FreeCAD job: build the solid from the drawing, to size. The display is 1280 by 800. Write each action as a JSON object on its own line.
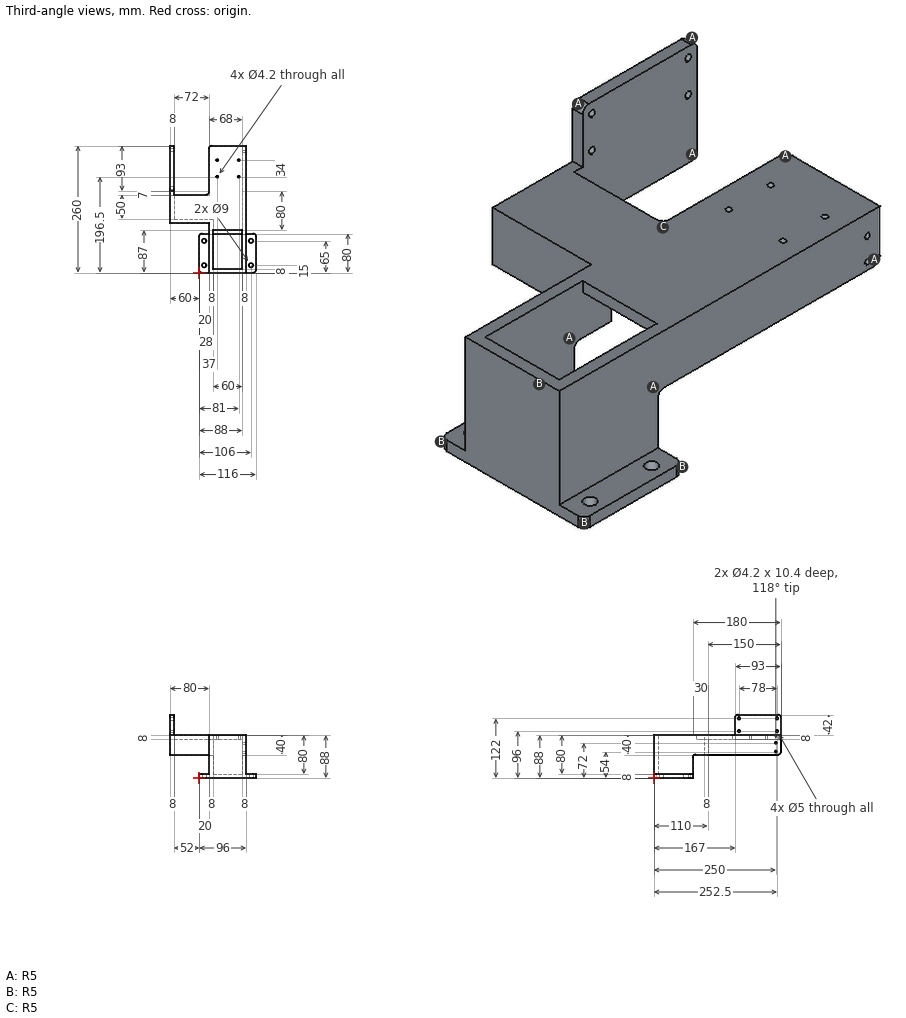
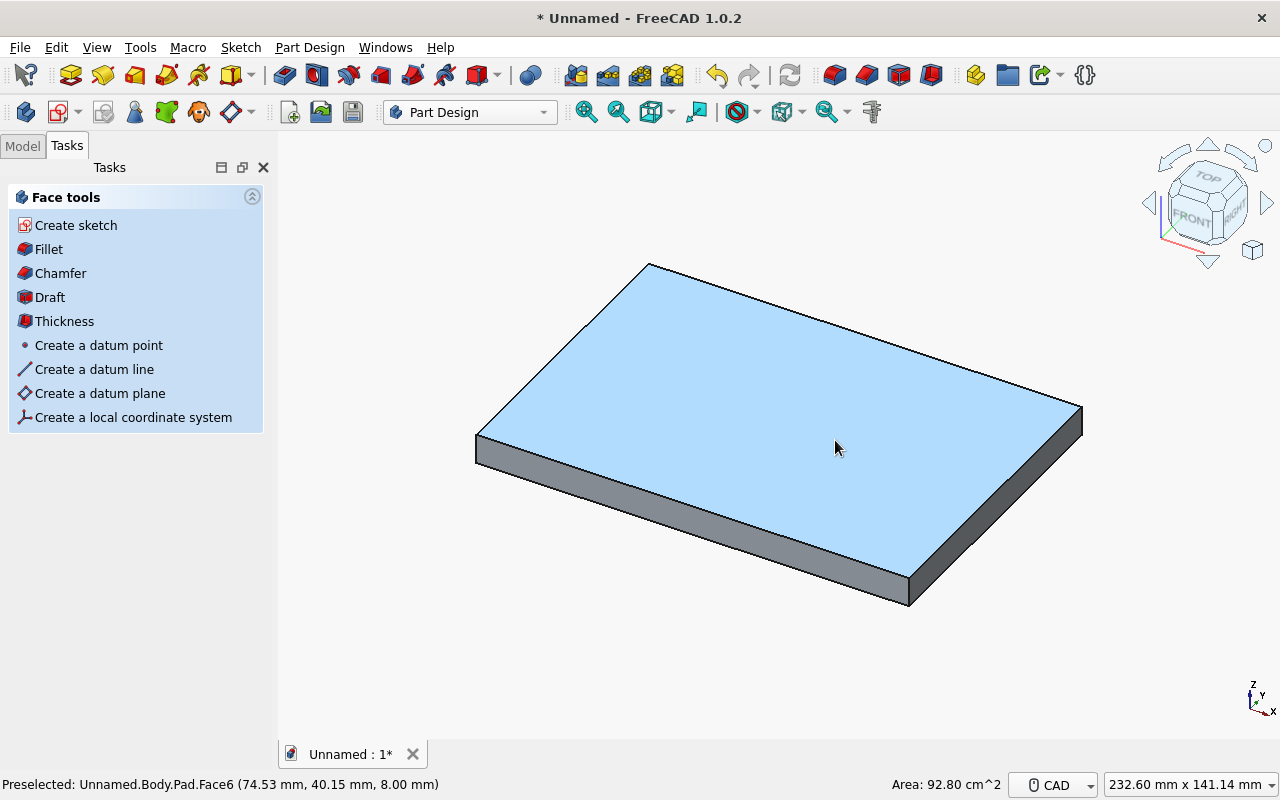
{"action": "left_click", "coordinate": [58, 112]}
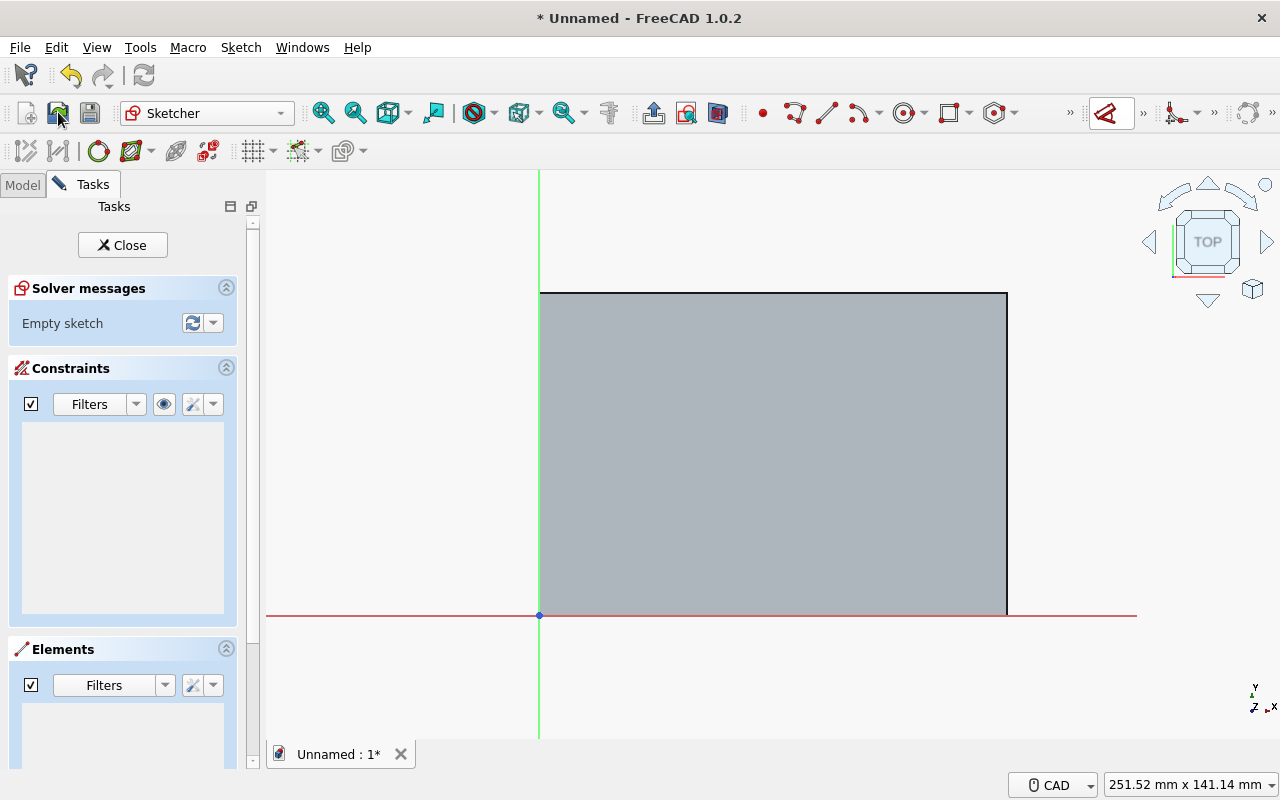
{"action": "left_click", "coordinate": [950, 114]}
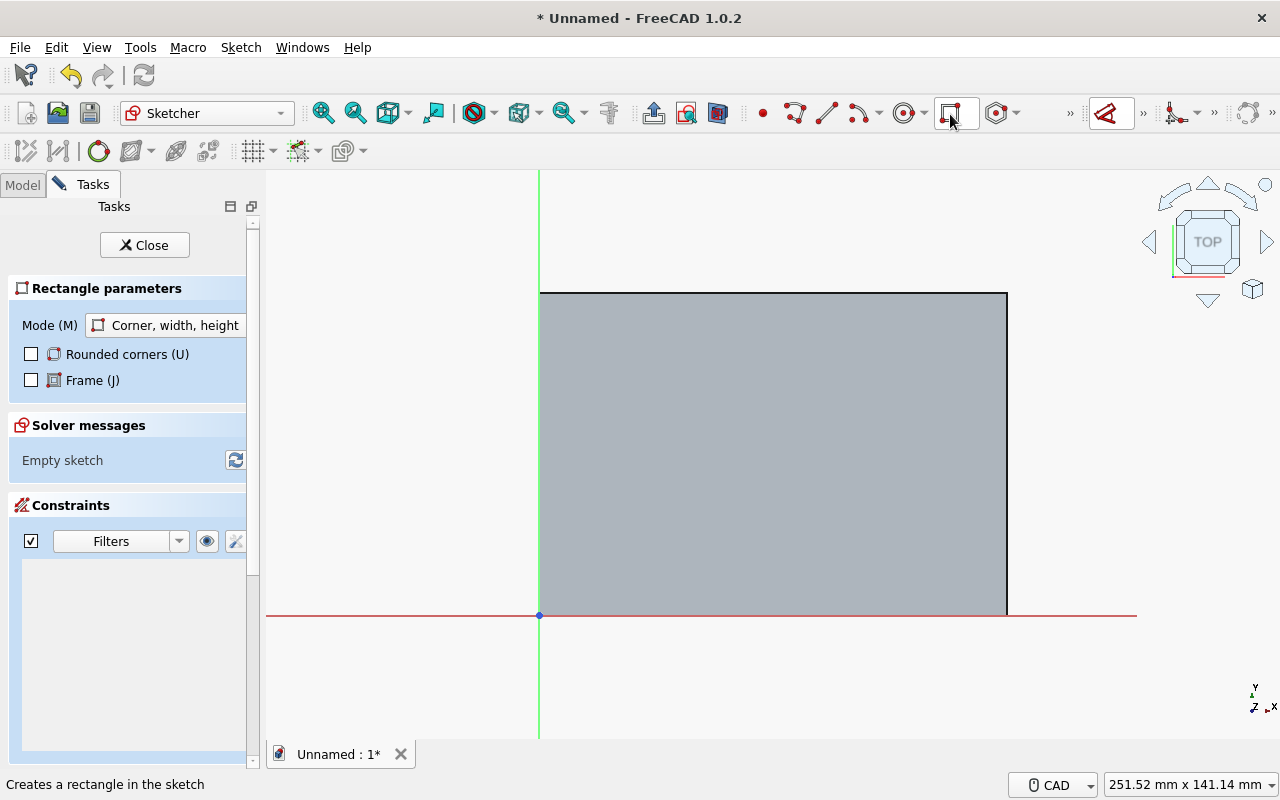
{"action": "left_click", "coordinate": [620, 293]}
{"action": "left_click", "coordinate": [652, 616]}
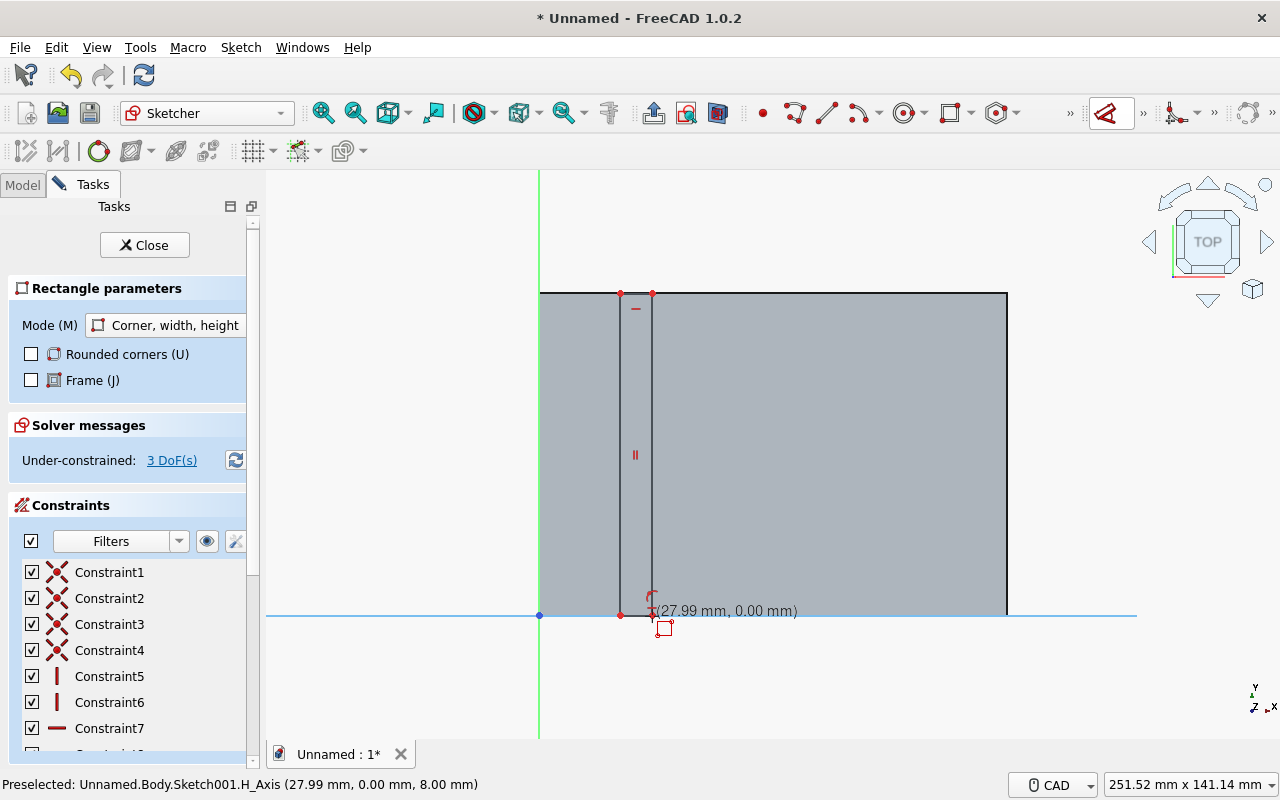
{"action": "left_click", "coordinate": [894, 293]}
{"action": "left_click", "coordinate": [926, 616]}
{"action": "key", "text": "Escape"}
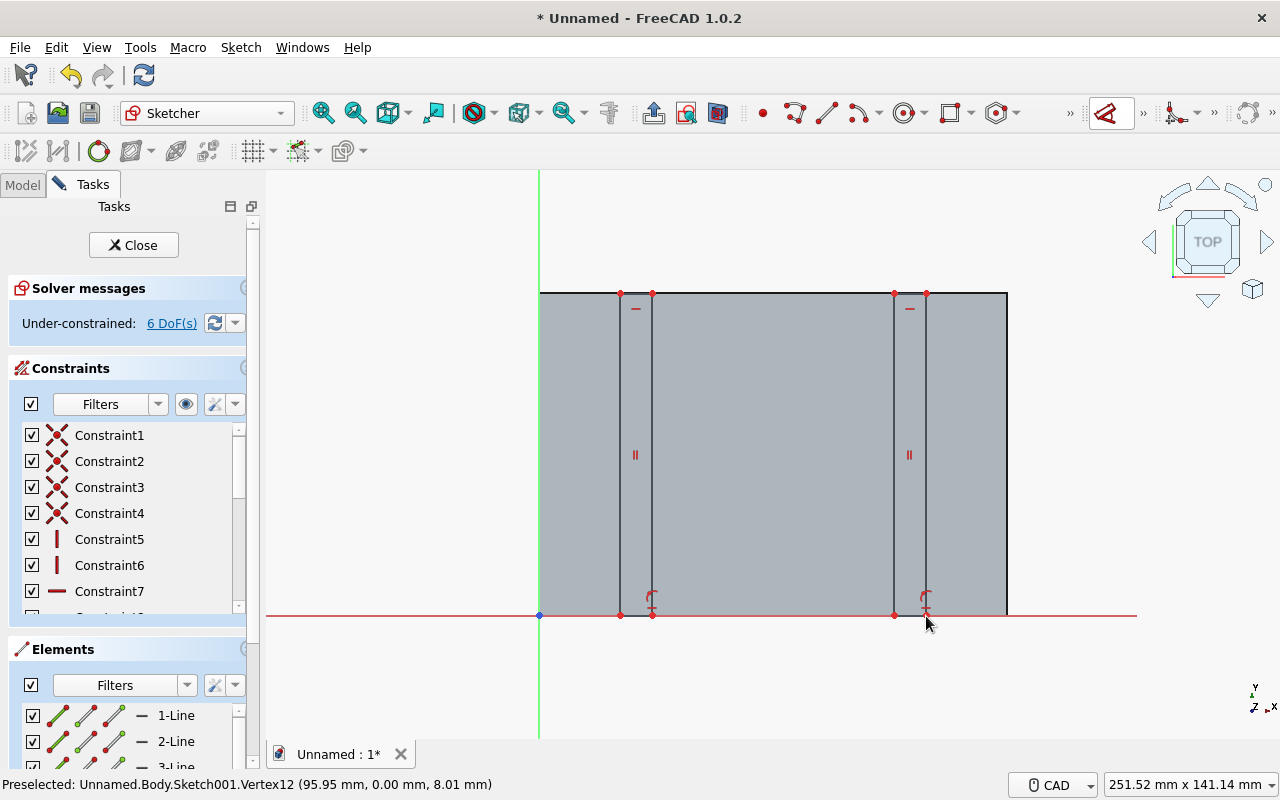
{"action": "scroll", "coordinate": [630, 616], "scroll_direction": "up", "scroll_amount": 2}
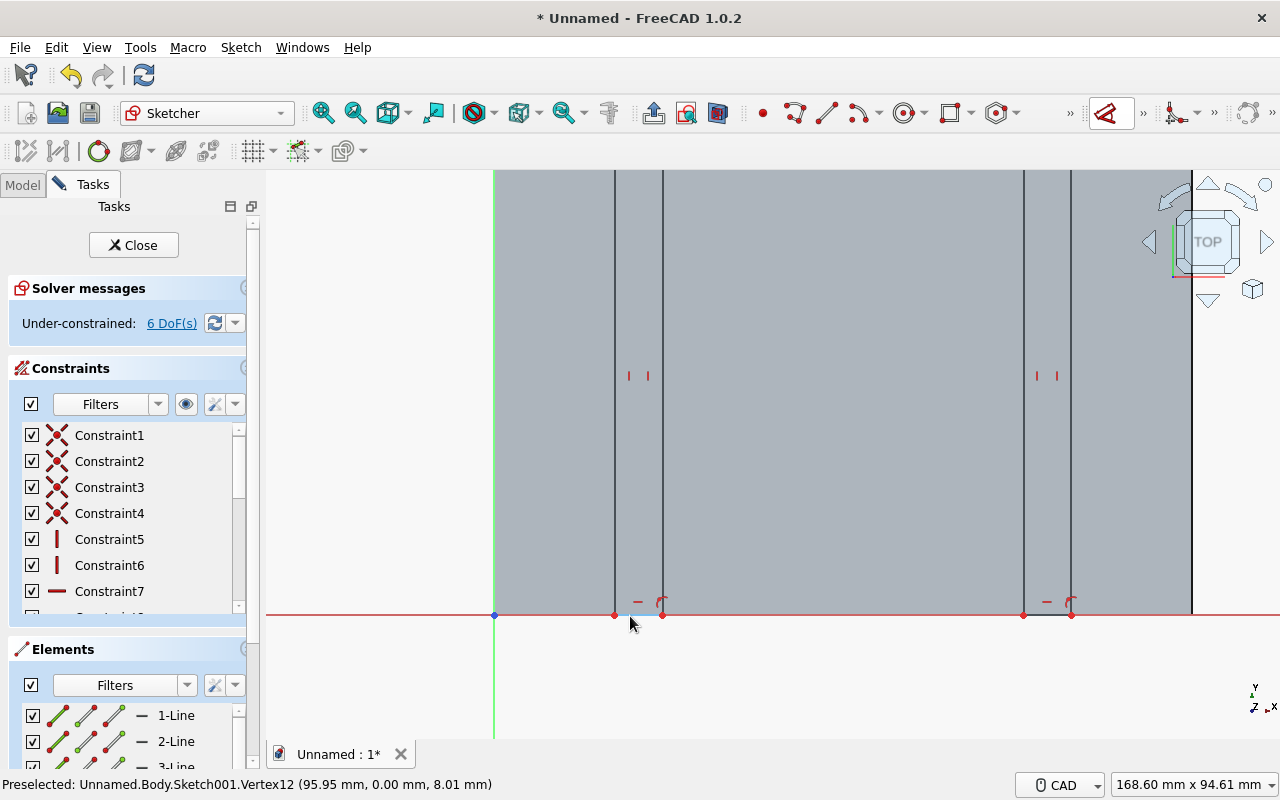
{"action": "left_click", "coordinate": [629, 615]}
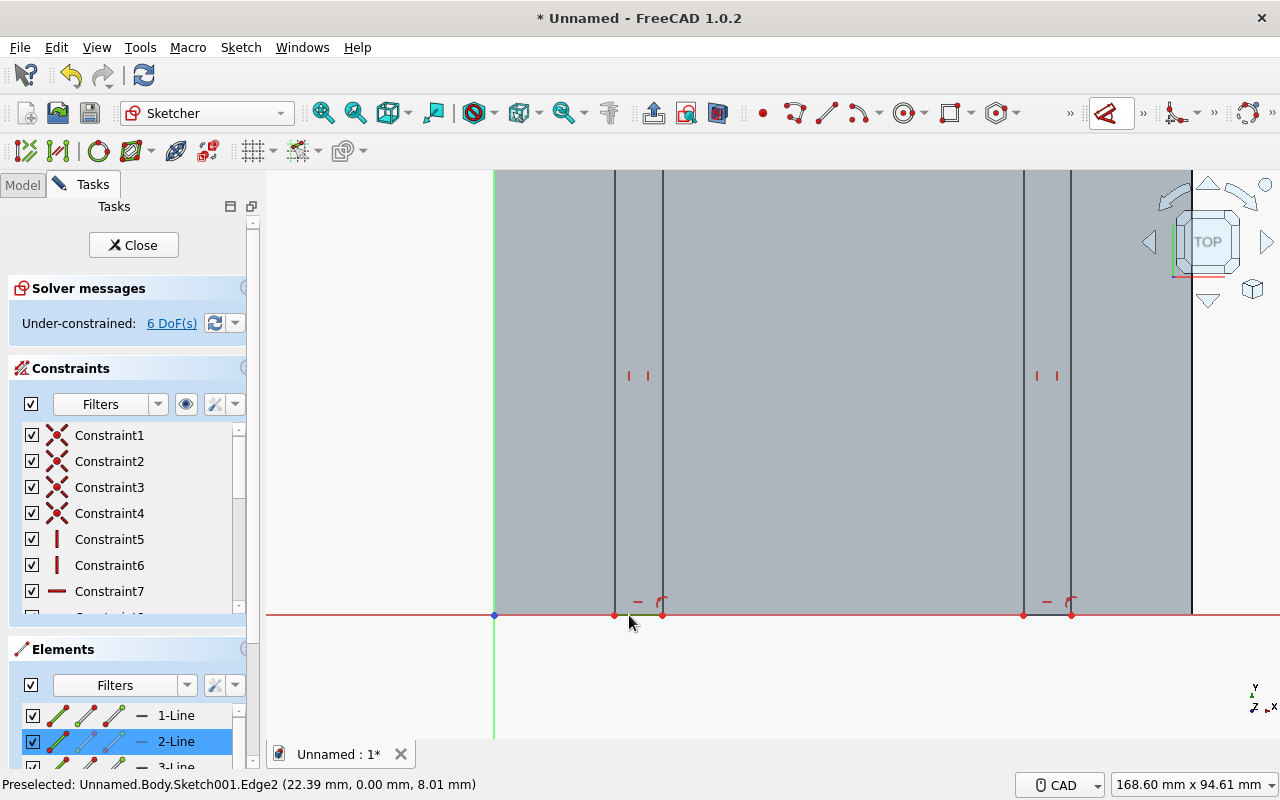
{"action": "left_click", "coordinate": [1128, 114]}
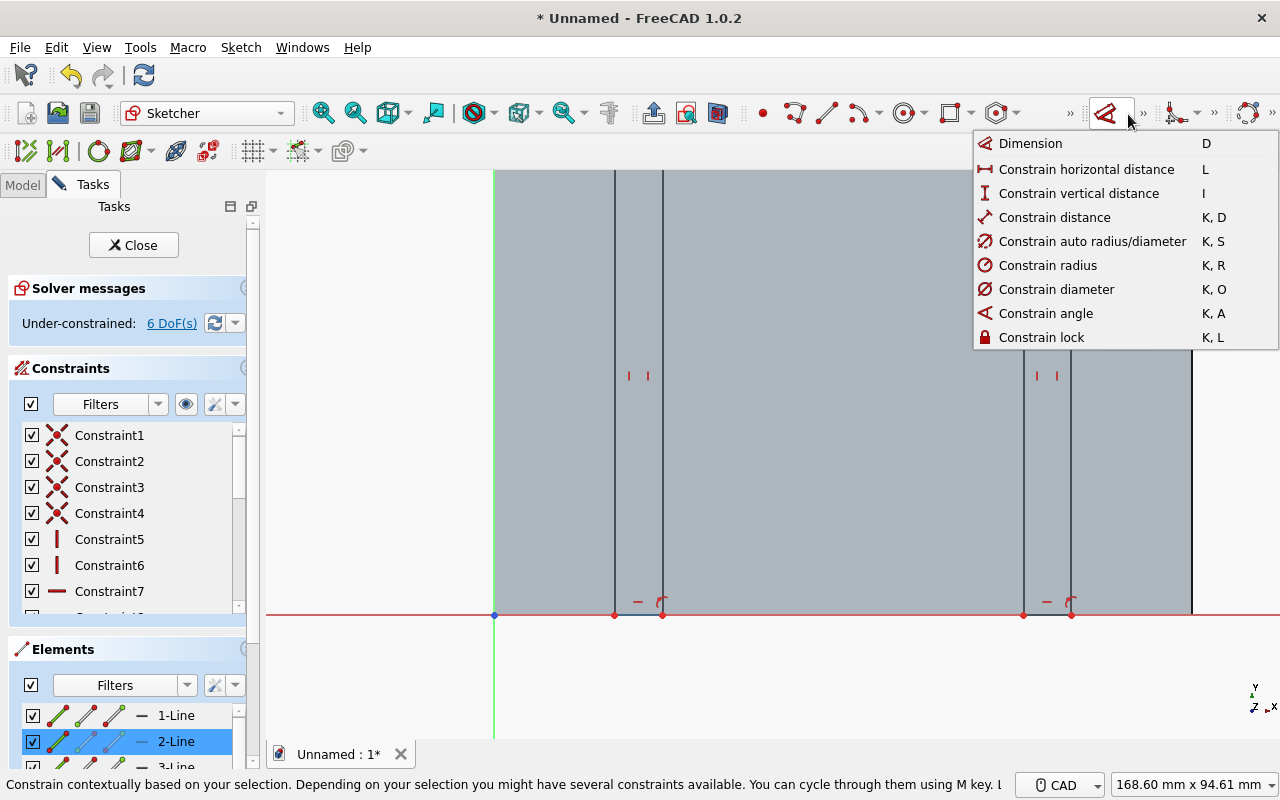
{"action": "left_click", "coordinate": [1126, 169]}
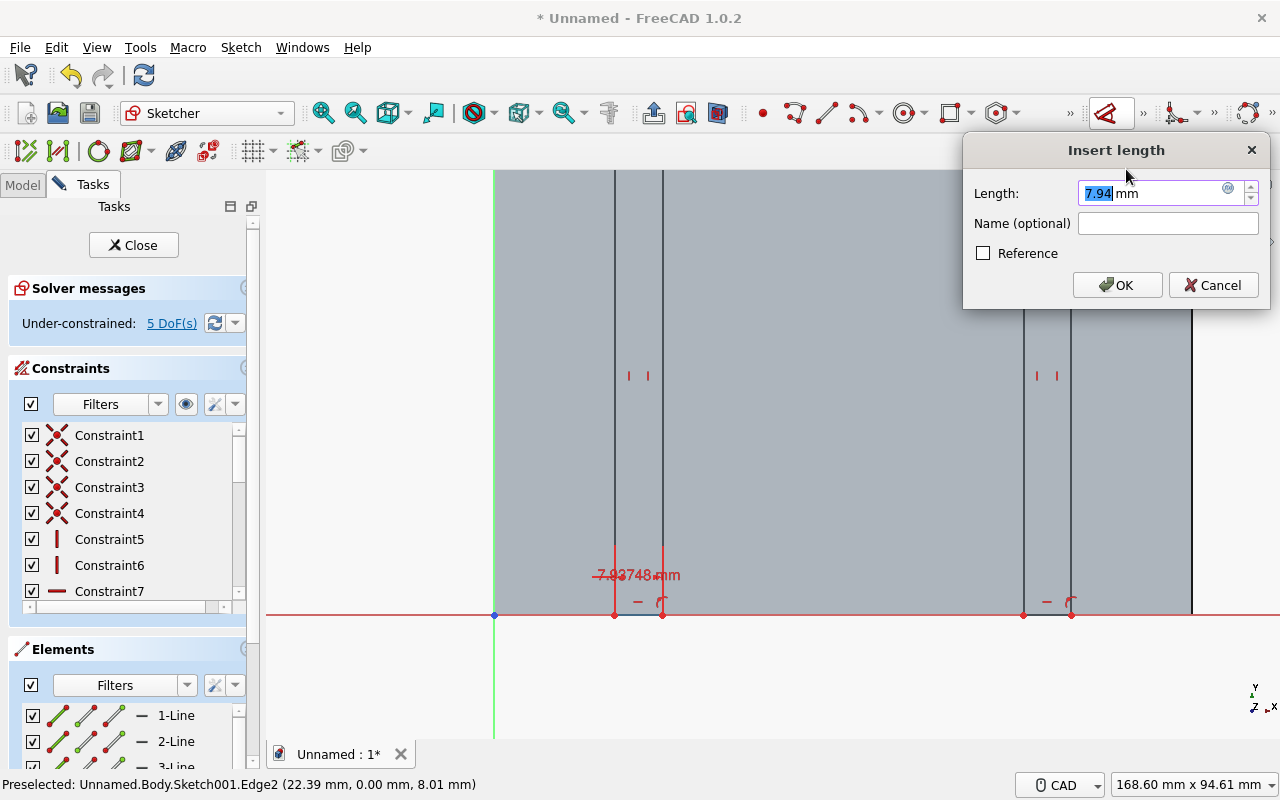
{"action": "type", "text": "8"}
{"action": "key", "text": "Return"}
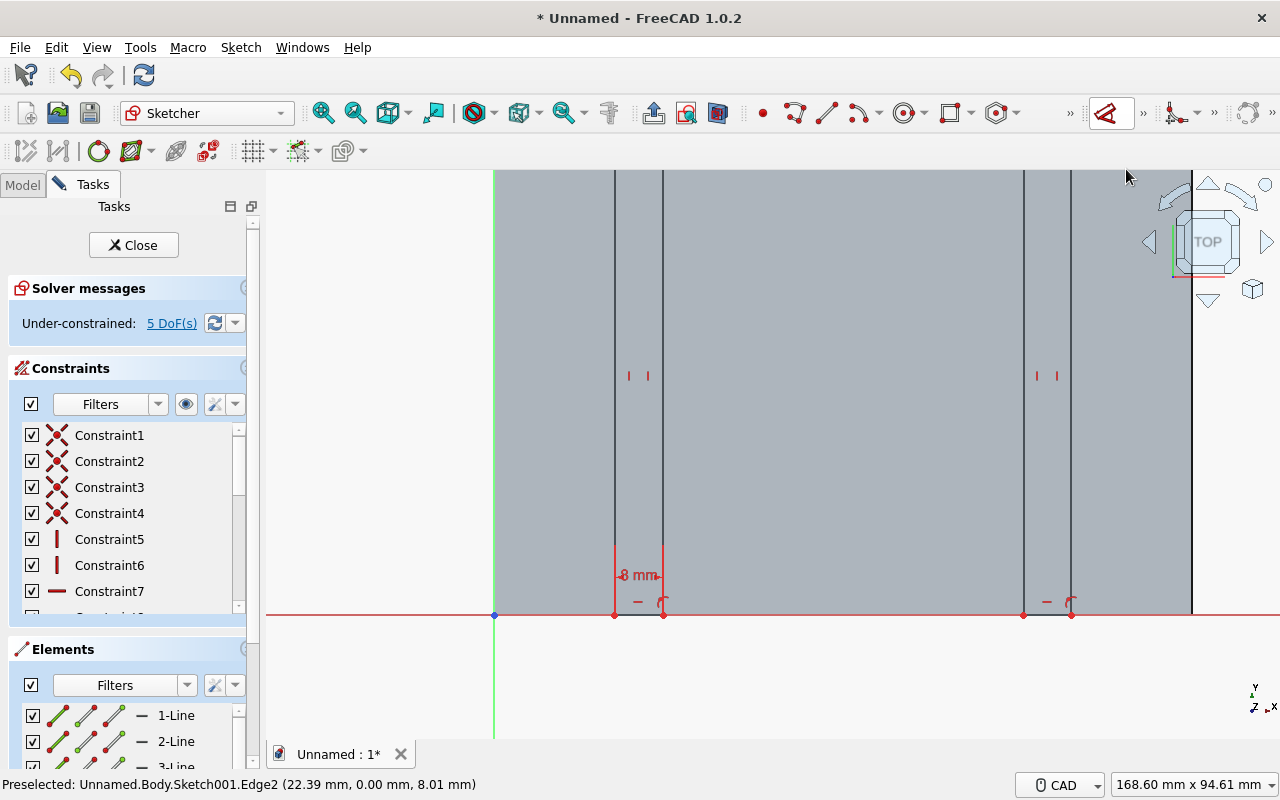
{"action": "left_click", "coordinate": [1038, 615]}